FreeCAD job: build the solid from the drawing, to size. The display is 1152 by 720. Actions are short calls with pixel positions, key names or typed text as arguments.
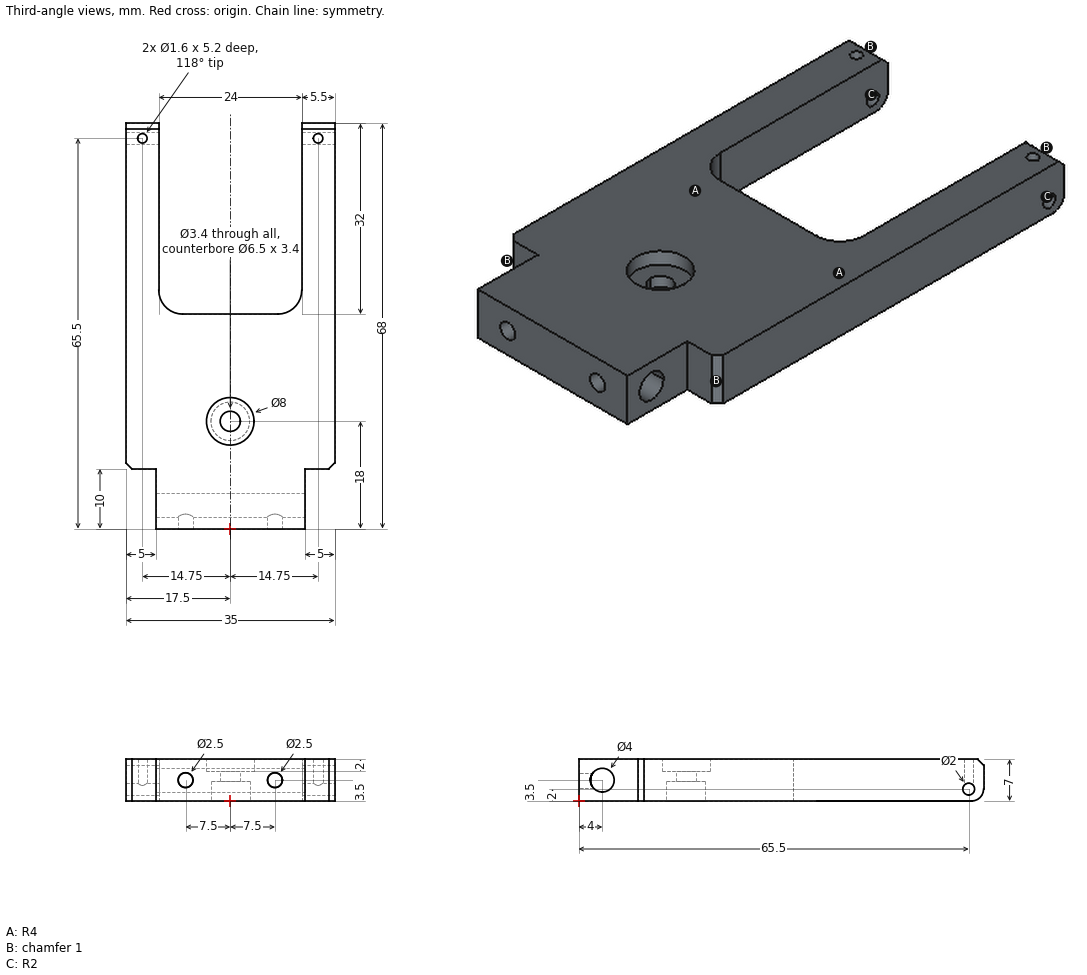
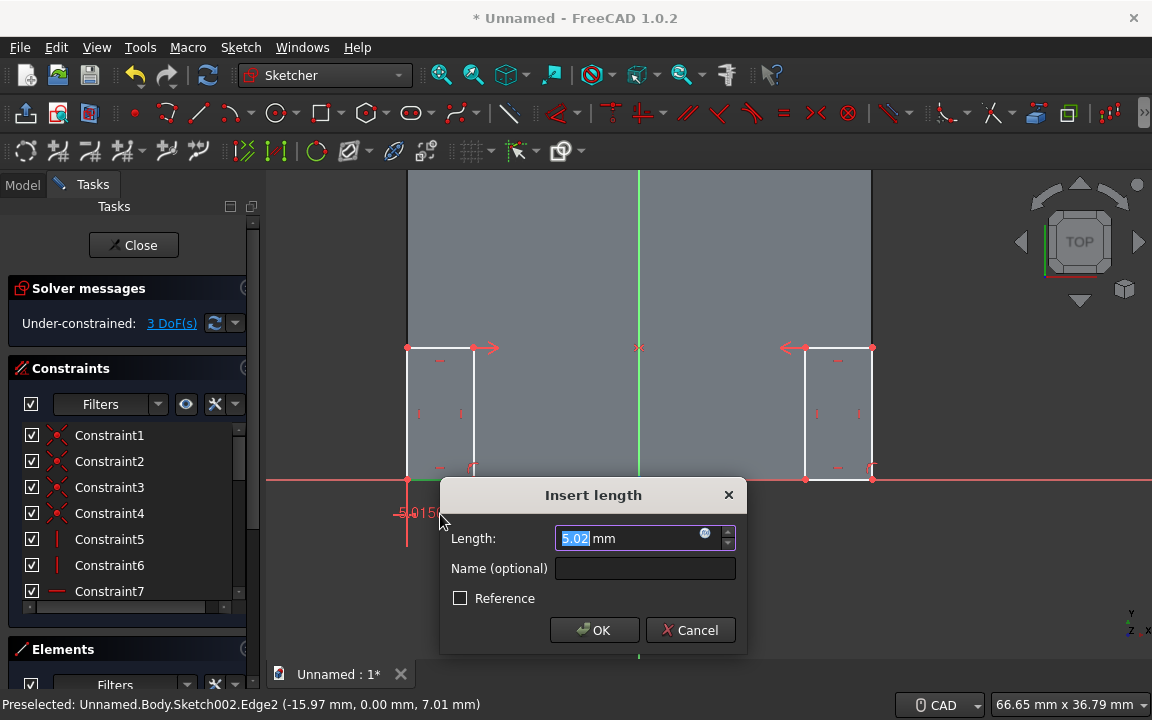
text(5)
key(Return)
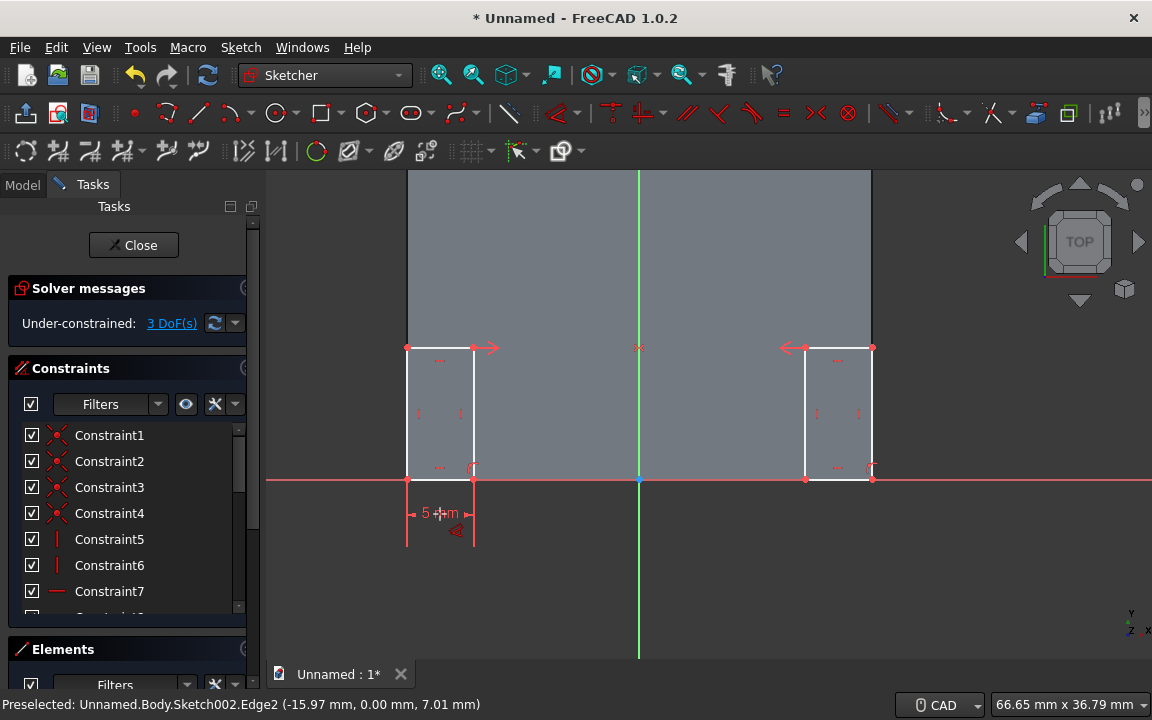
click(825, 480)
click(838, 514)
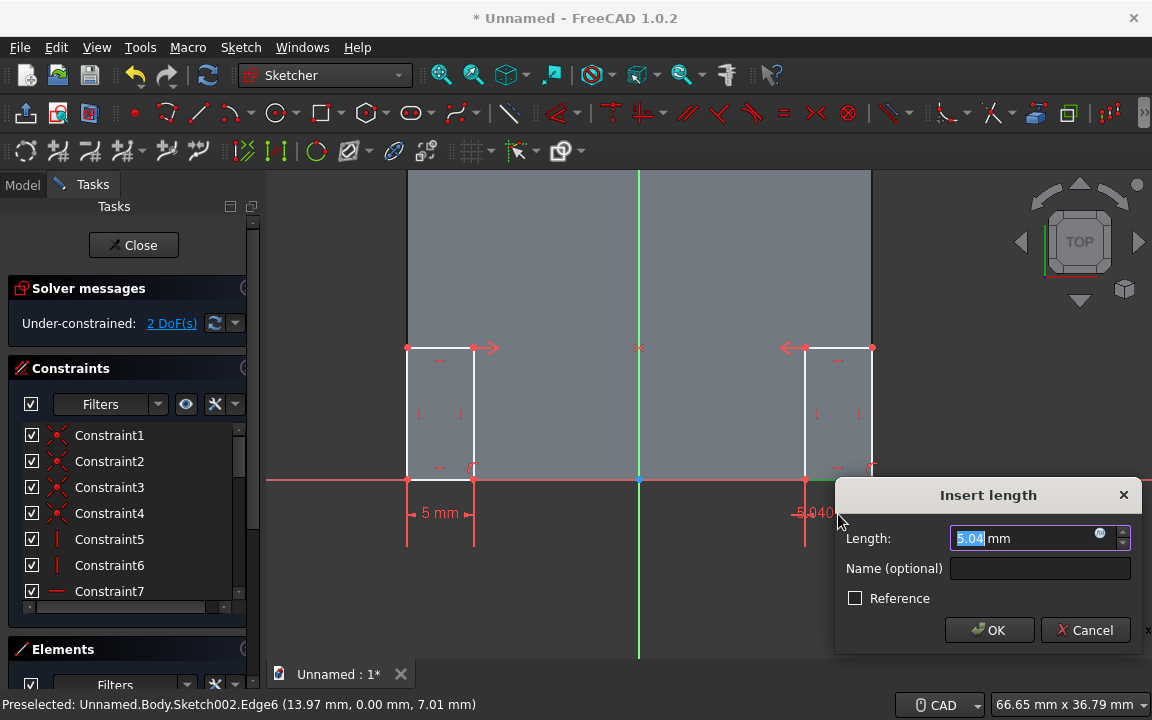
text(5)
key(Return)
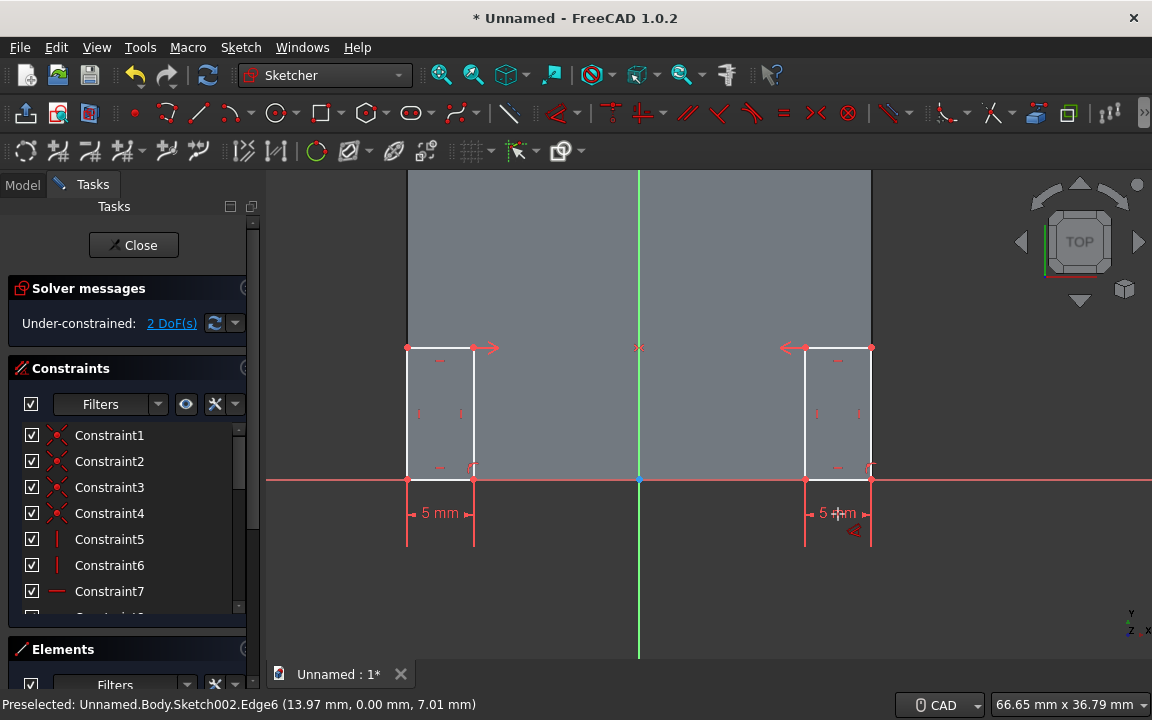
click(407, 388)
click(373, 414)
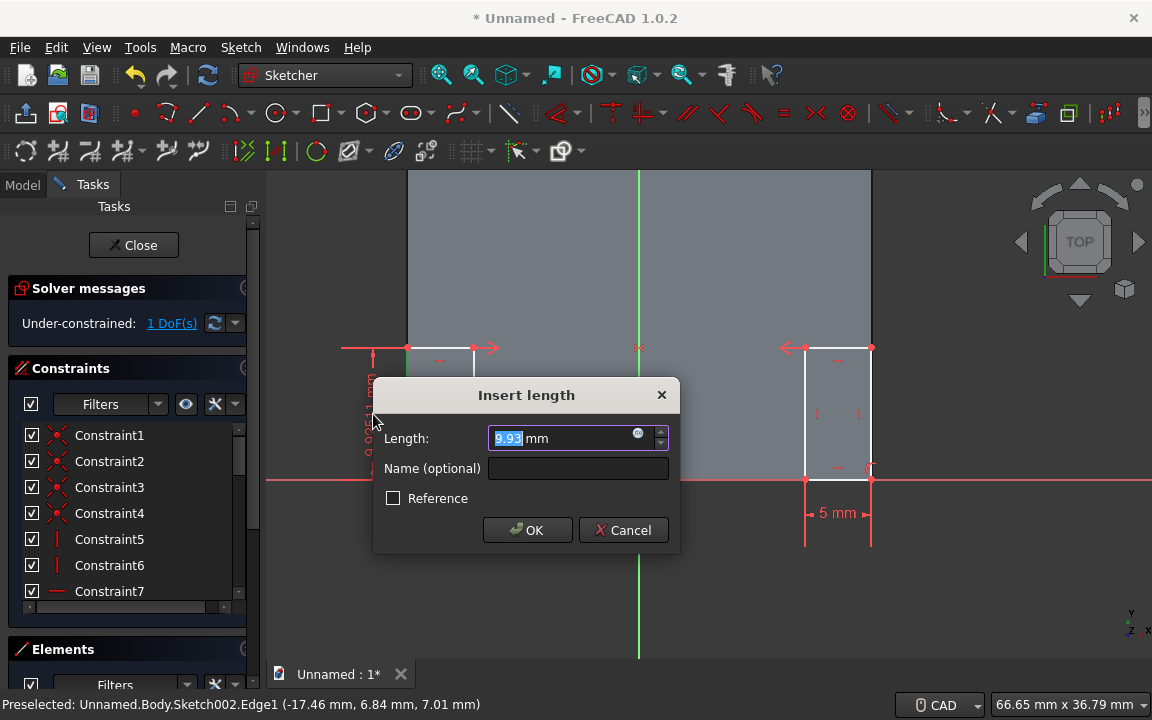
text(10)
key(Return)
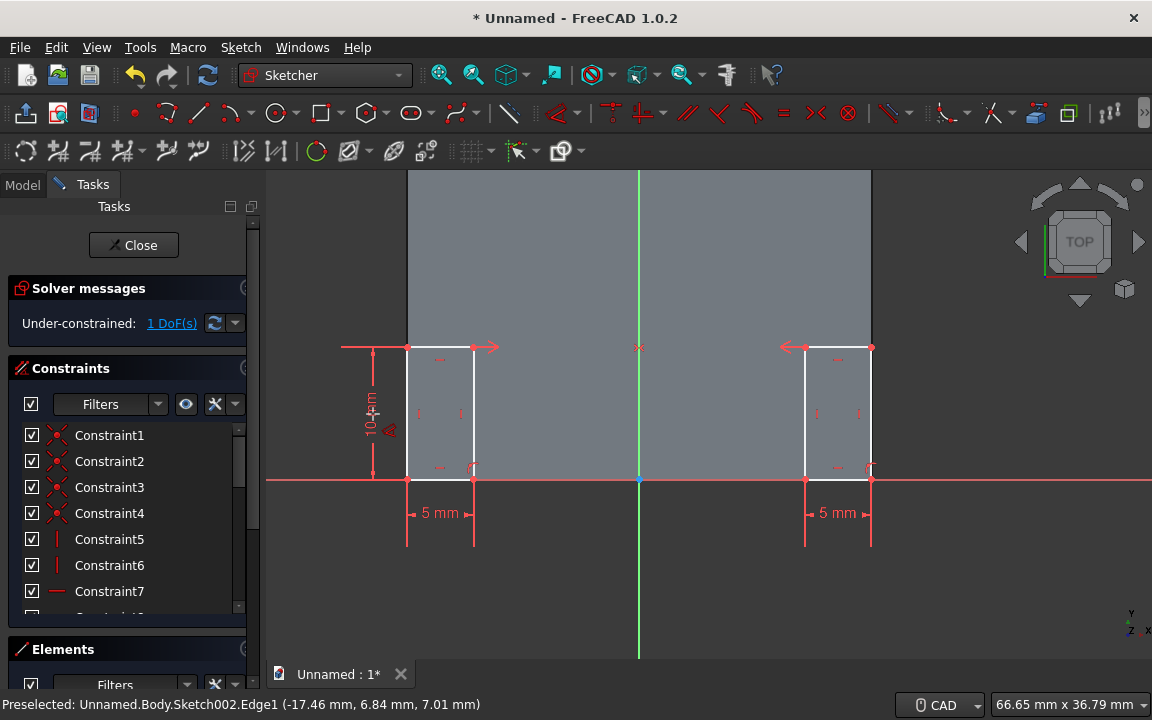
click(407, 347)
click(523, 514)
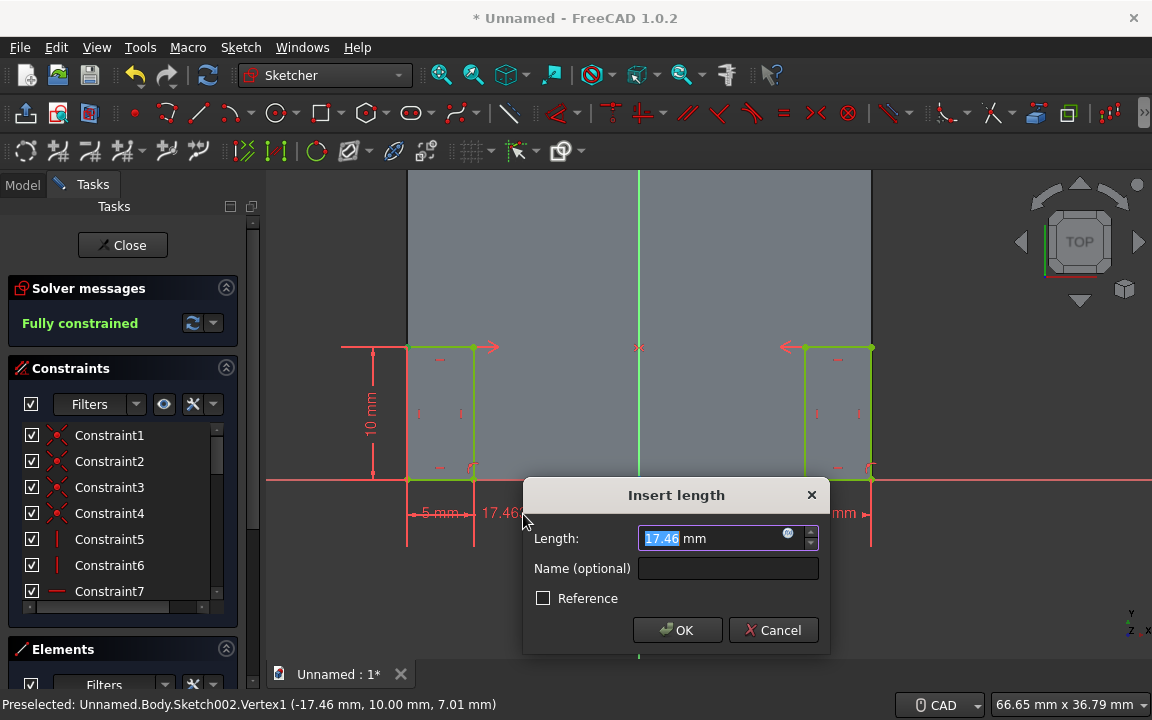
text(17.5)
key(Return)
key(Escape)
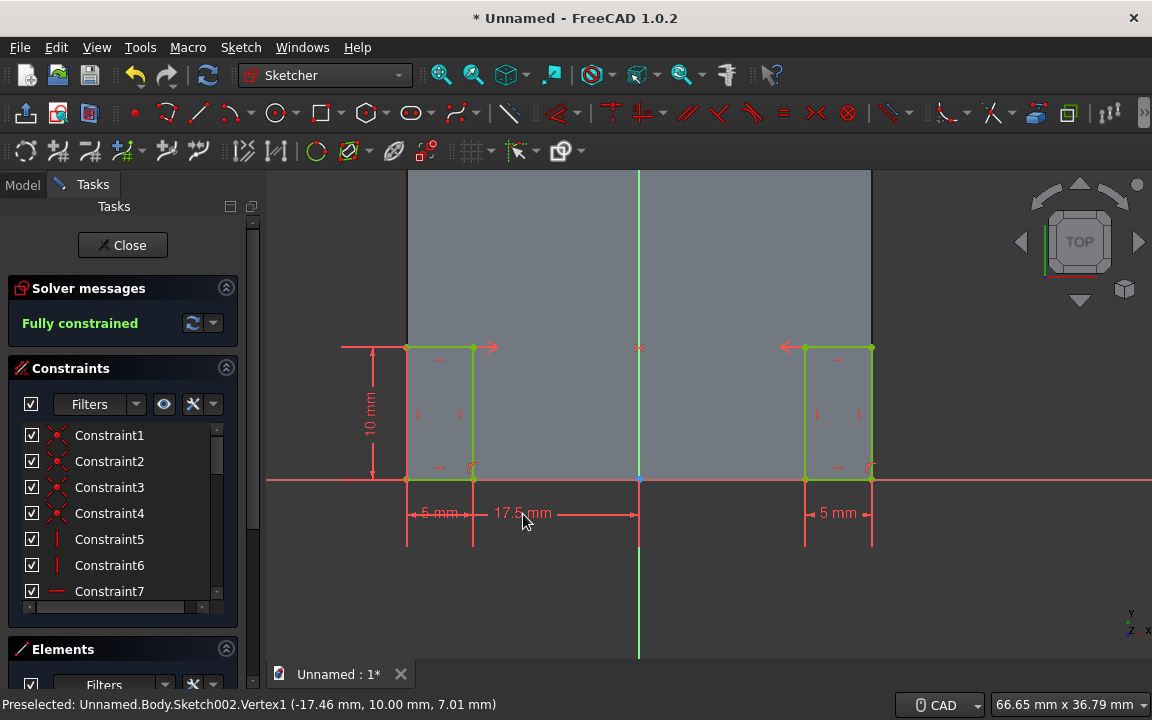
click(123, 245)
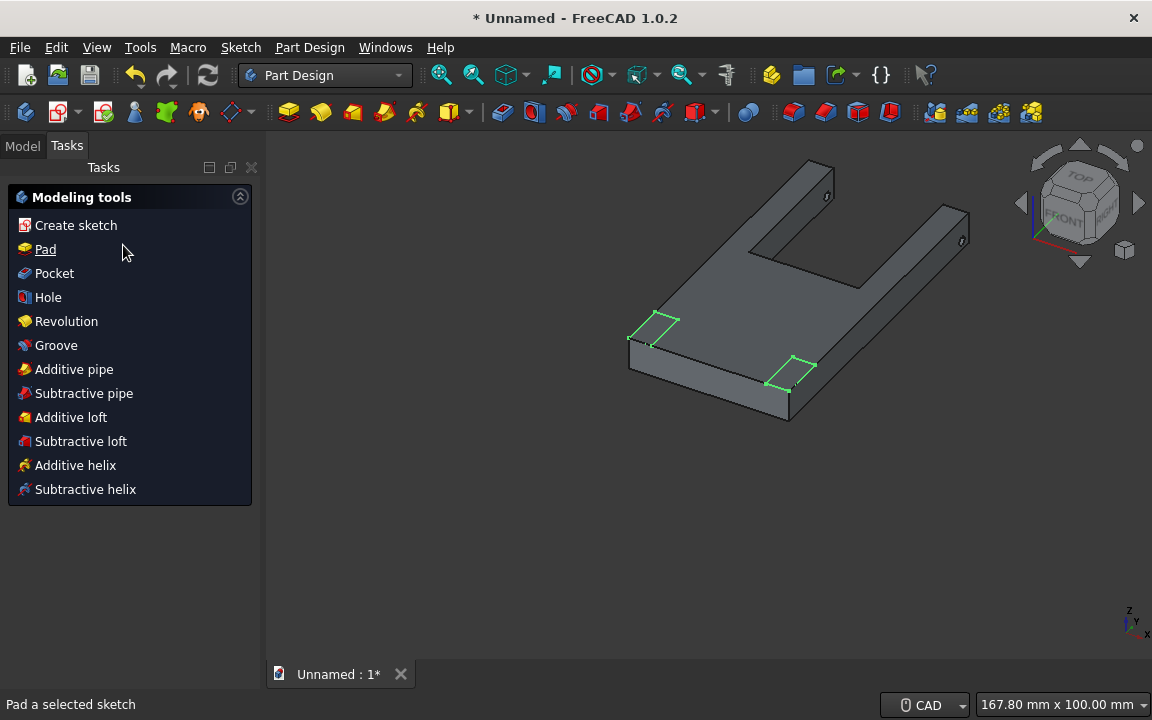
click(504, 112)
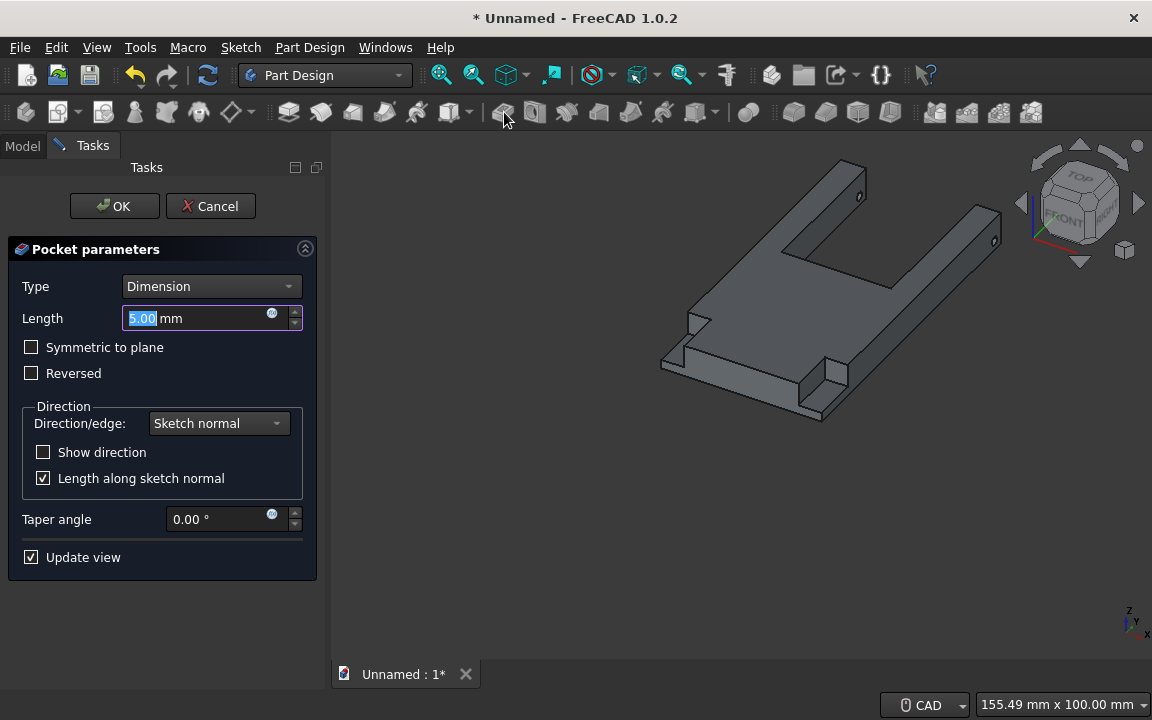
click(212, 286)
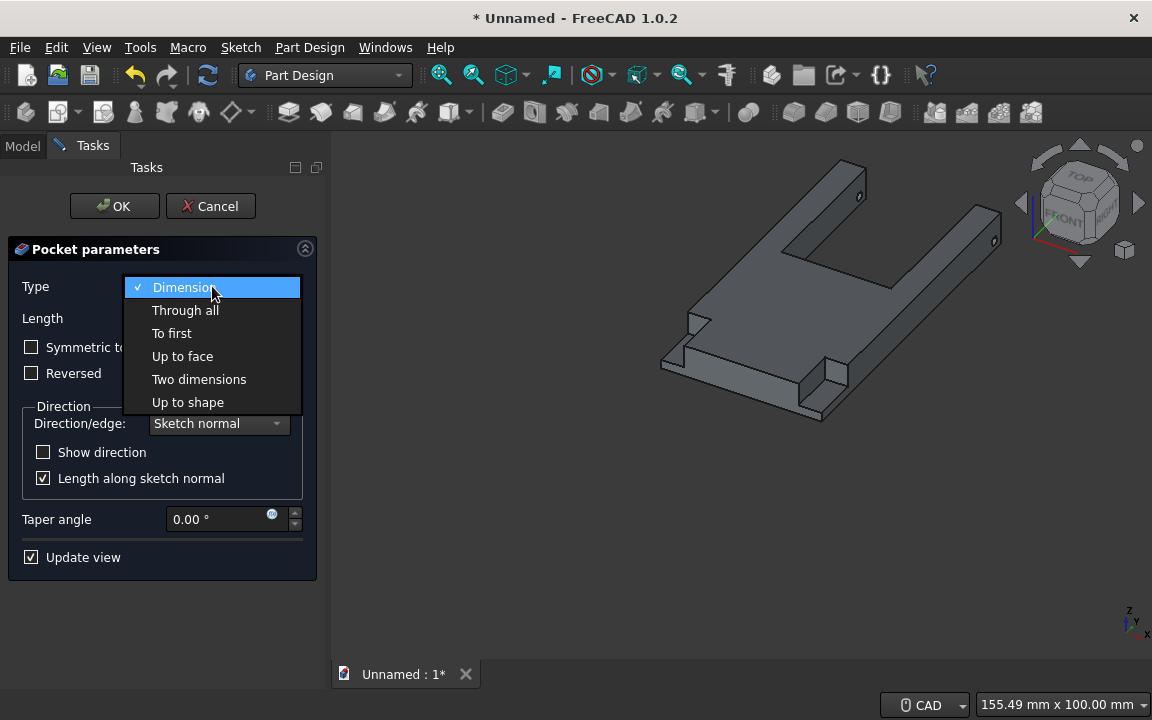
click(212, 310)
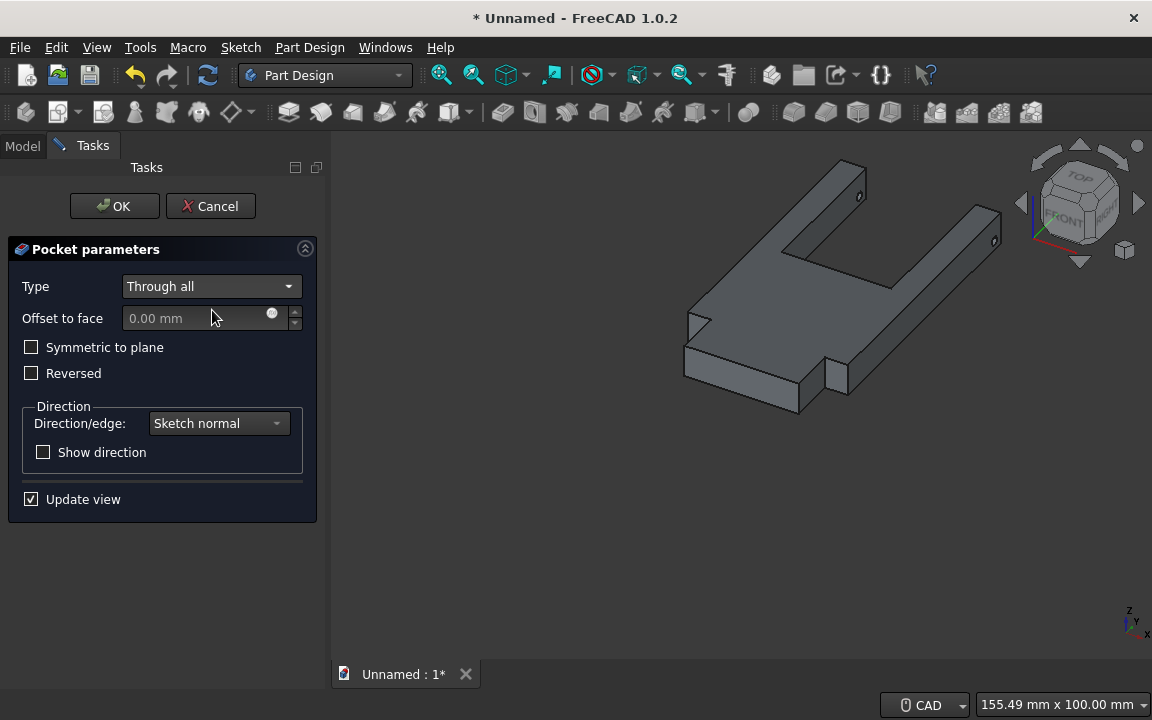
click(115, 206)